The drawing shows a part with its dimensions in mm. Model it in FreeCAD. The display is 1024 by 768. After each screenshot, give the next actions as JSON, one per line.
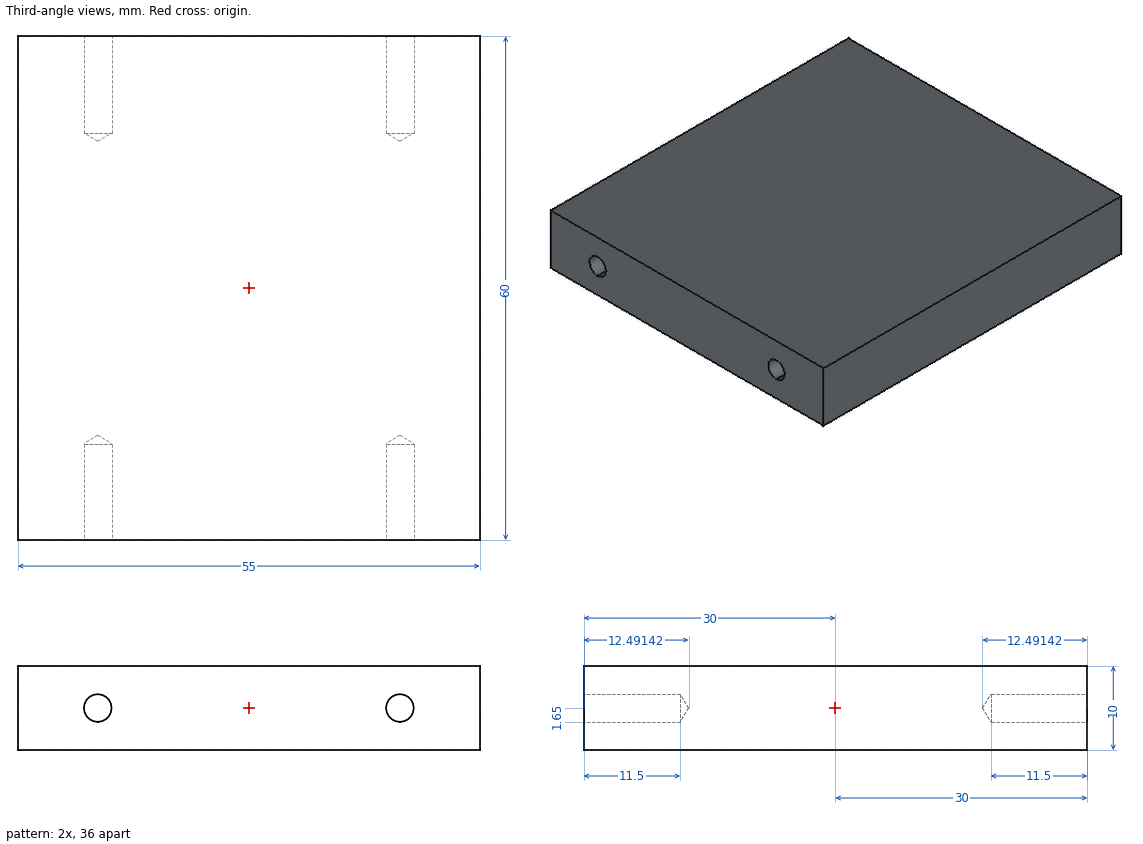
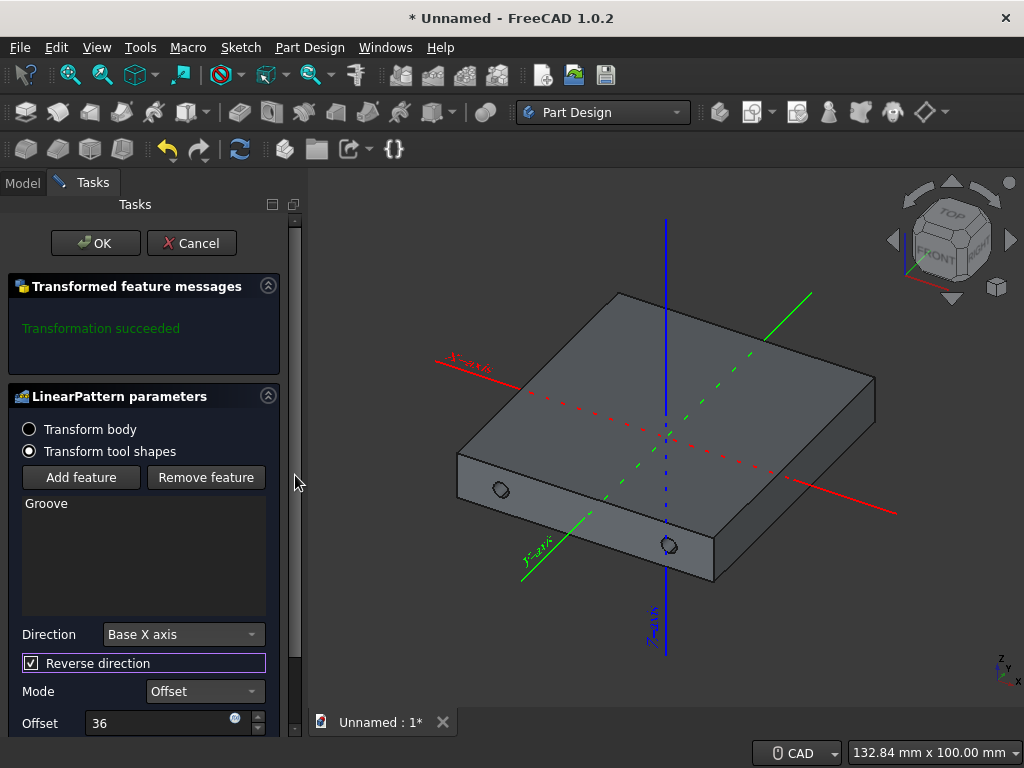
{"action": "left_click", "coordinate": [96, 243]}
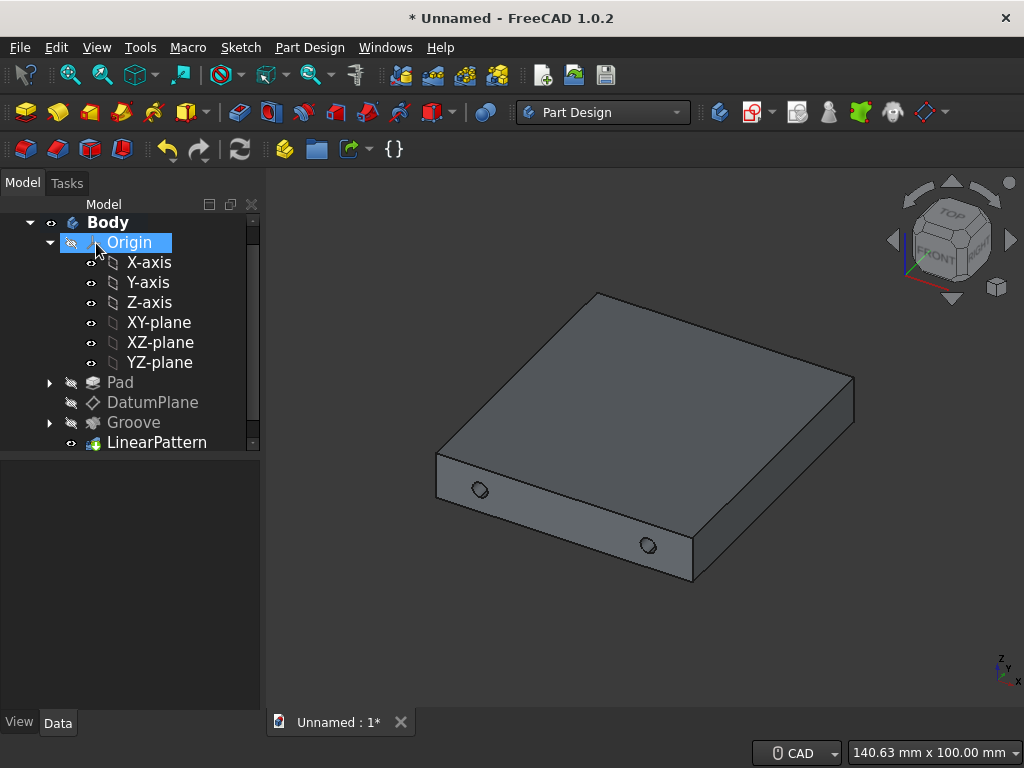
{"action": "left_click", "coordinate": [116, 423]}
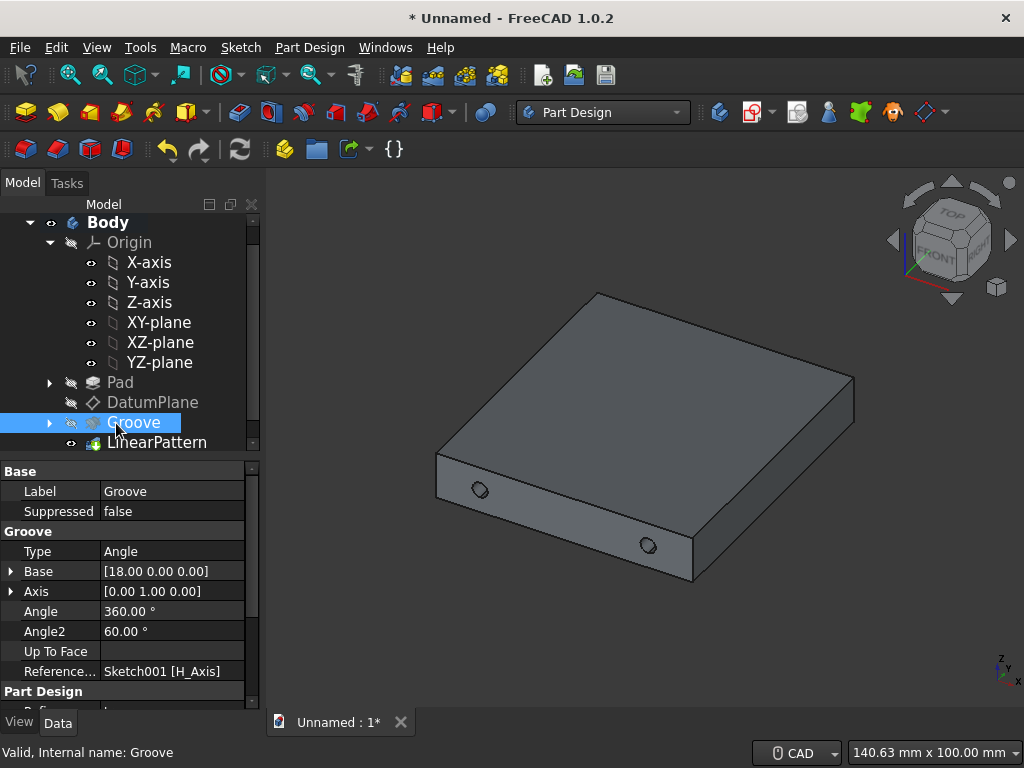
{"action": "left_click", "coordinate": [402, 76]}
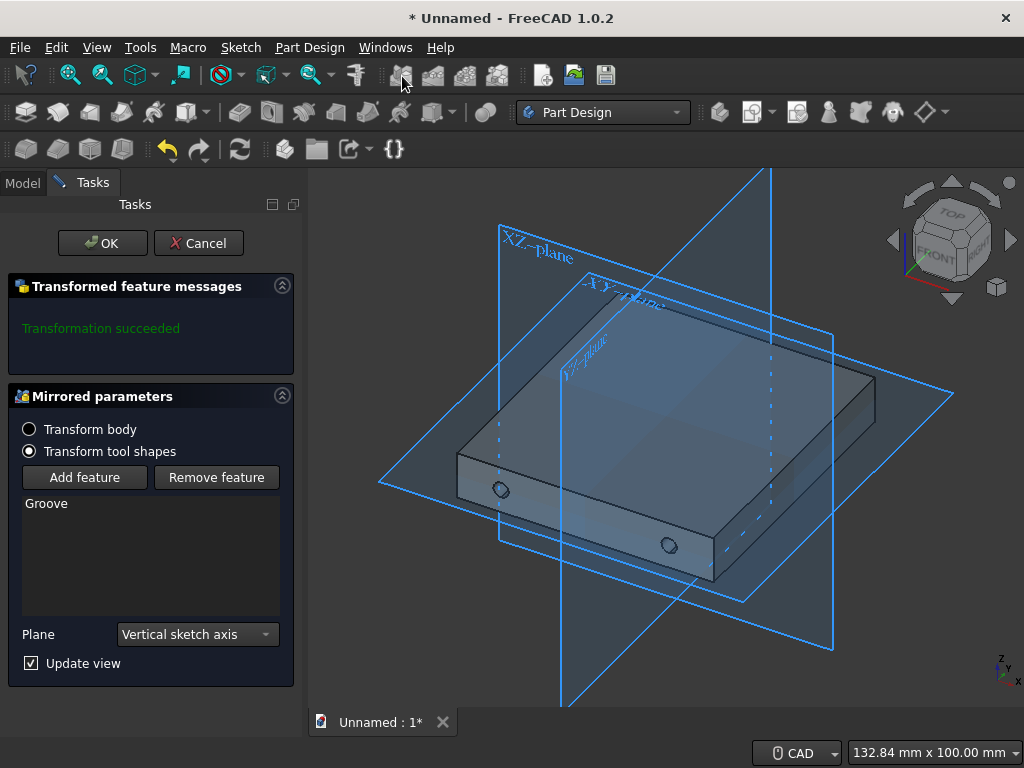
{"action": "left_click", "coordinate": [198, 634]}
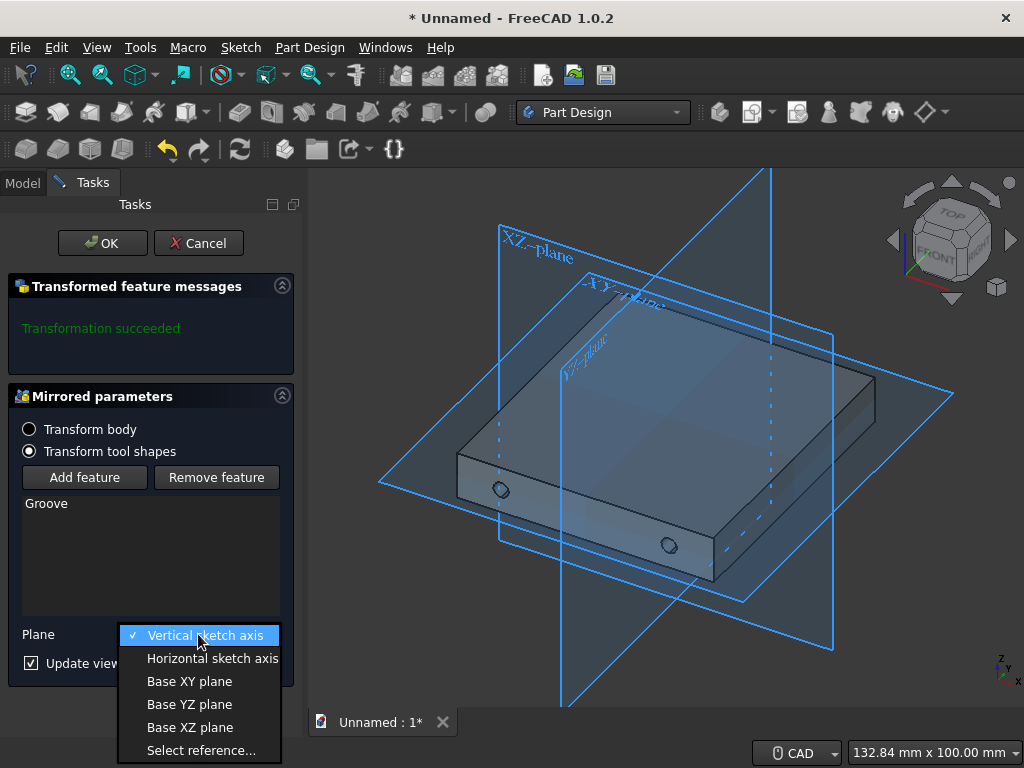
{"action": "left_click", "coordinate": [198, 728]}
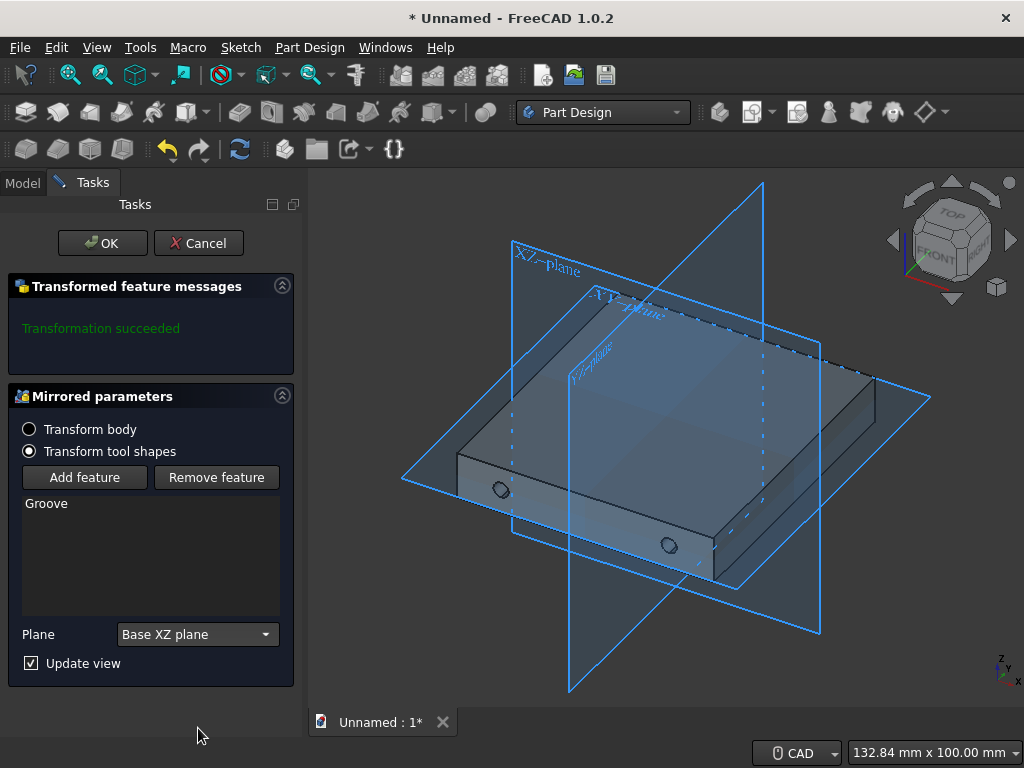
{"action": "left_click", "coordinate": [103, 243]}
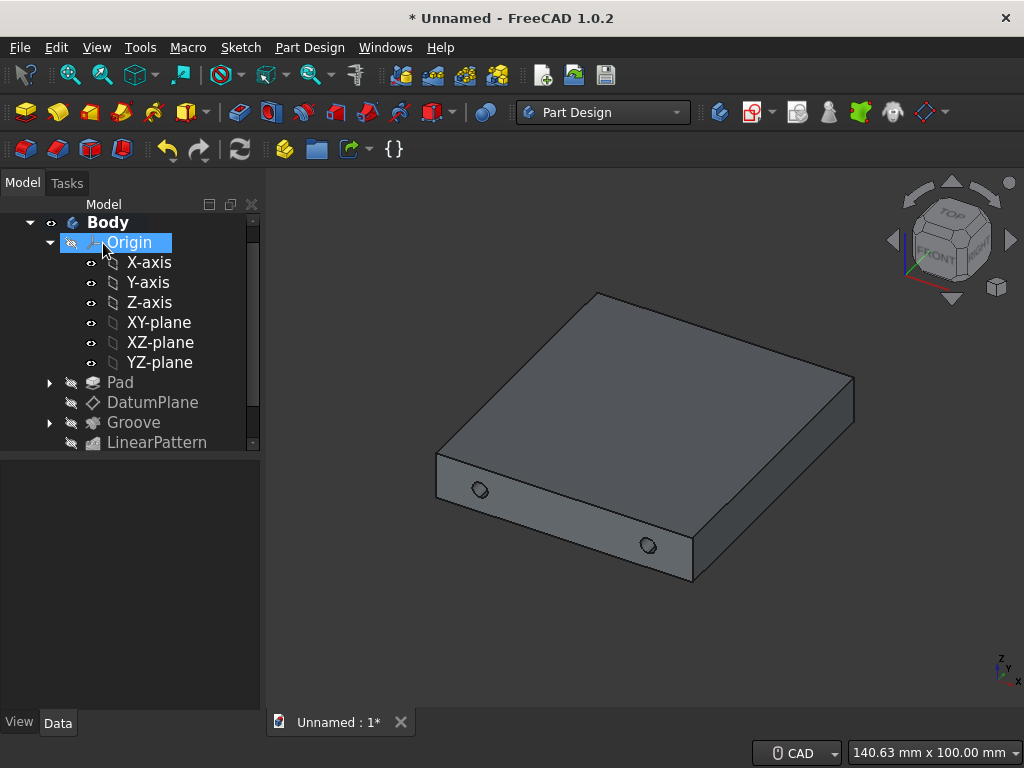
{"action": "left_click", "coordinate": [136, 363]}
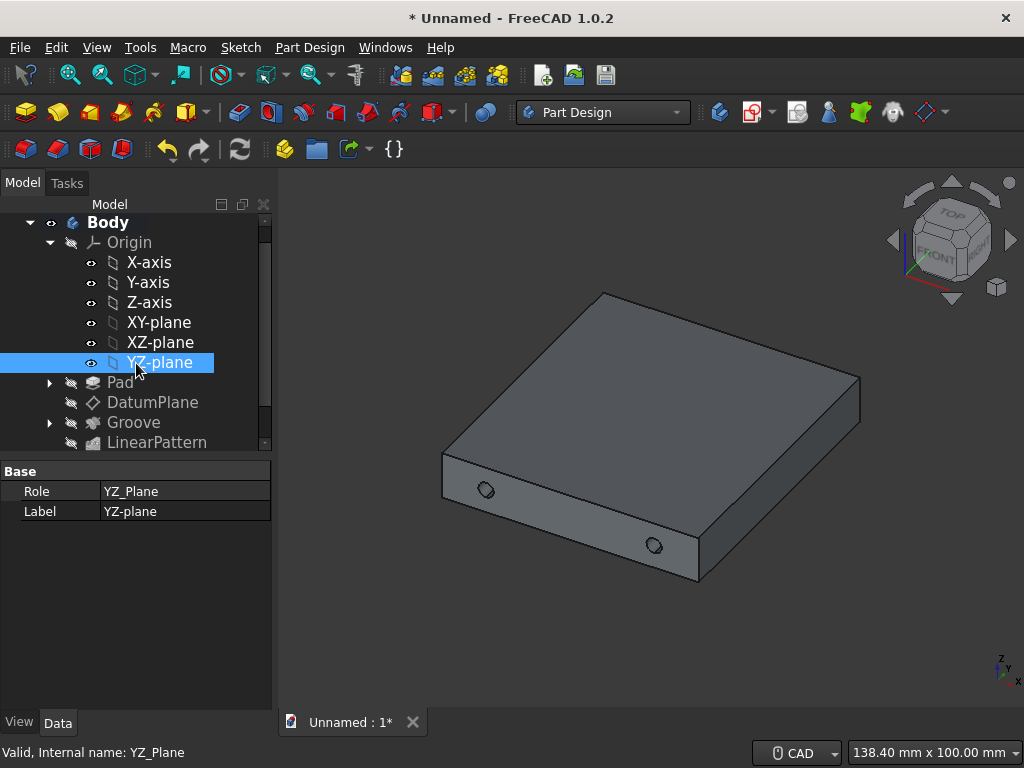
{"action": "left_click", "coordinate": [926, 112]}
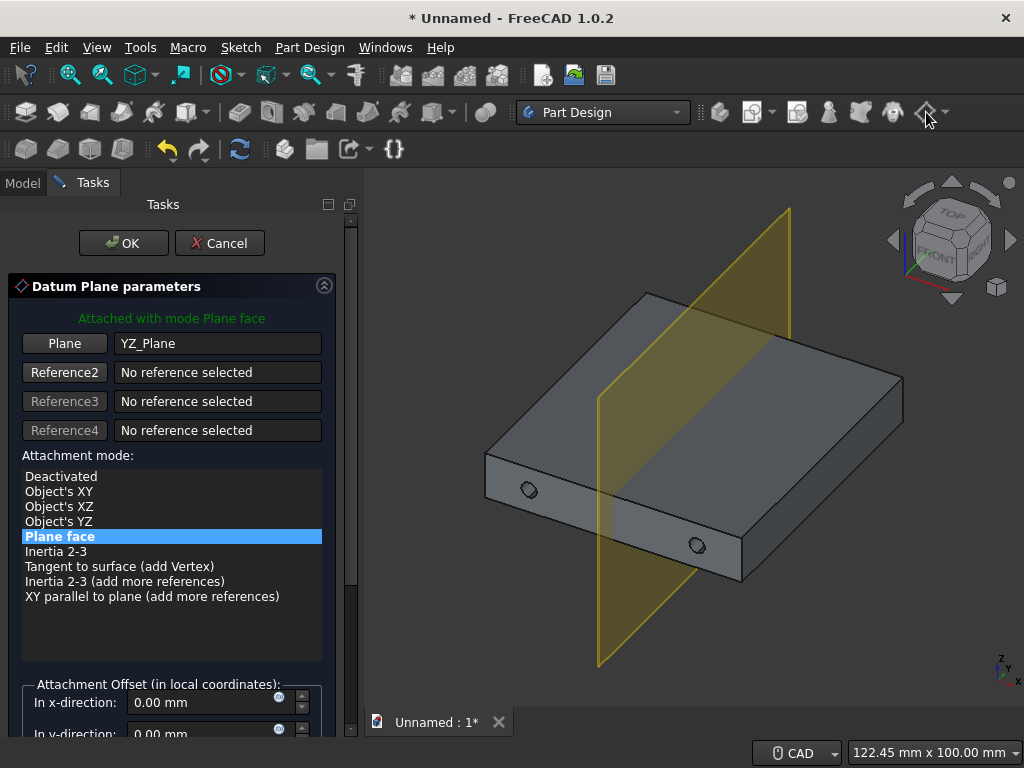
{"action": "scroll", "coordinate": [351, 475], "scroll_direction": "down", "scroll_amount": 2}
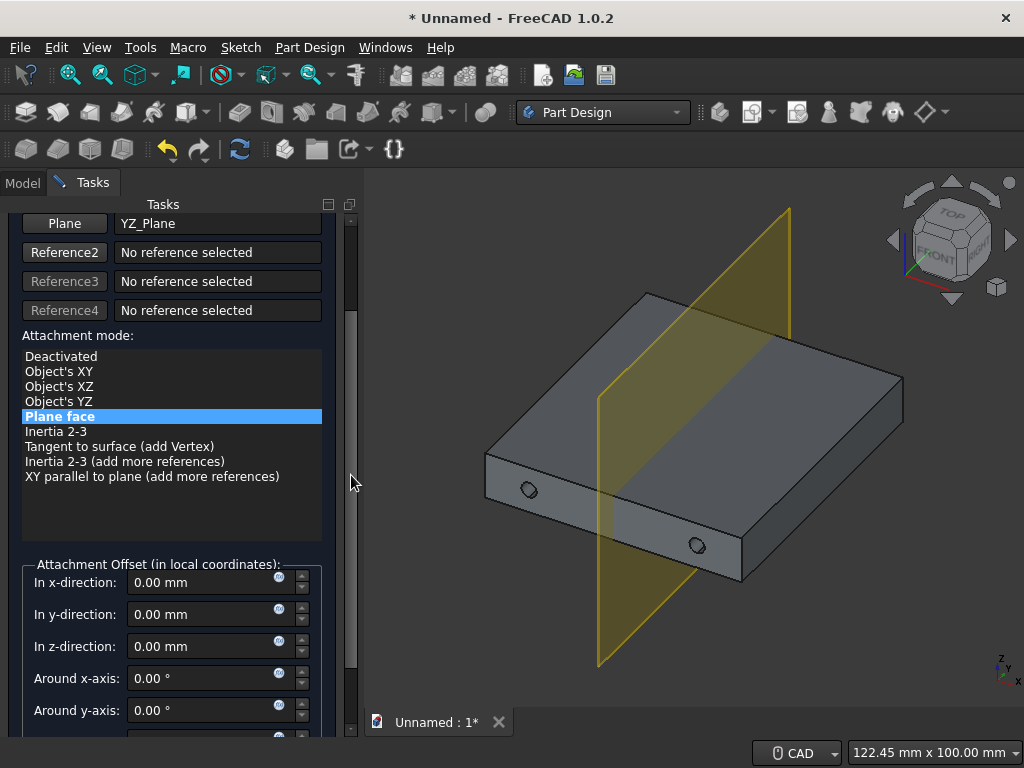
{"action": "triple_click", "coordinate": [210, 646]}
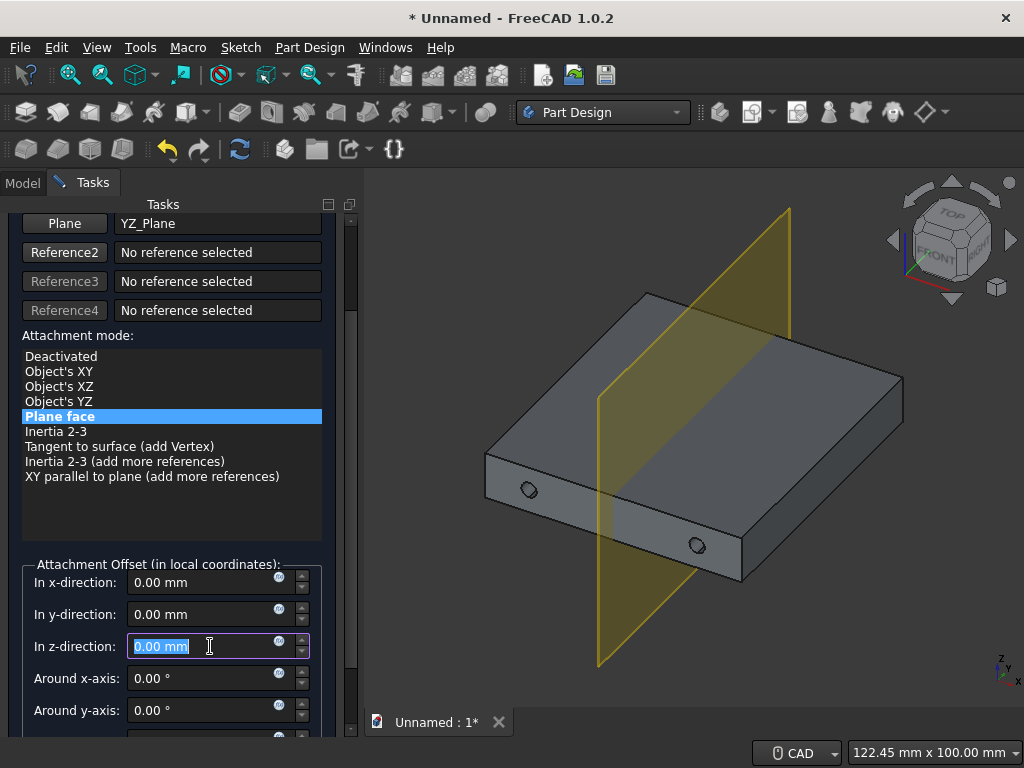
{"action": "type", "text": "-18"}
{"action": "key", "text": "Tab"}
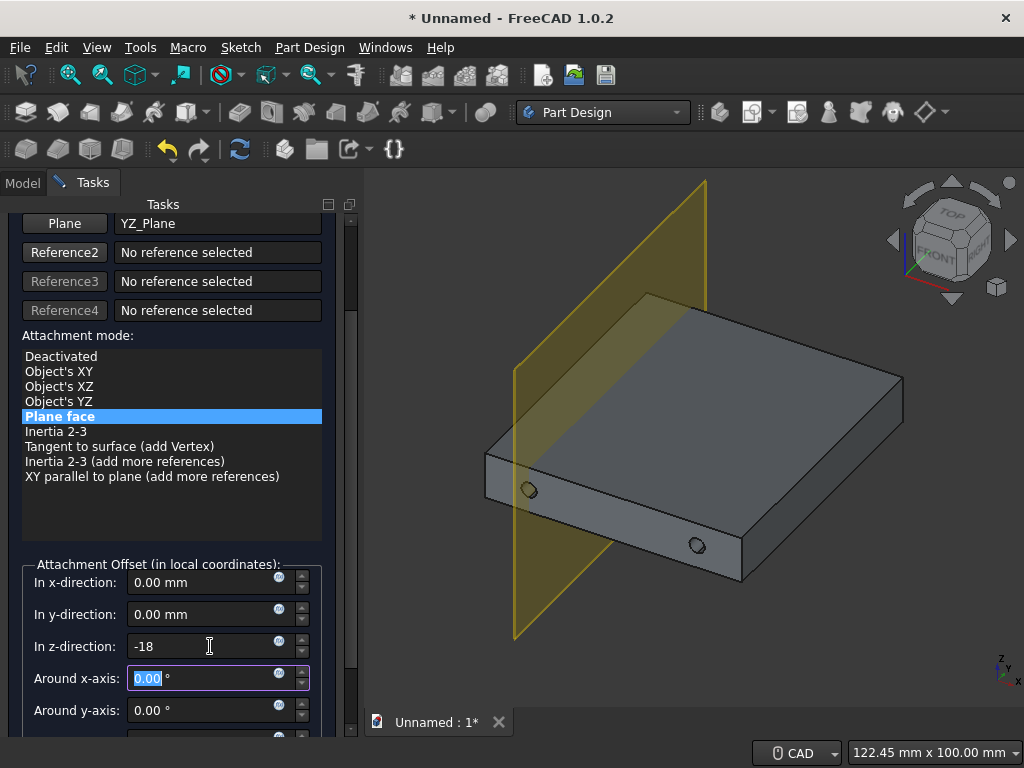
{"action": "scroll", "coordinate": [351, 475], "scroll_direction": "up", "scroll_amount": 3}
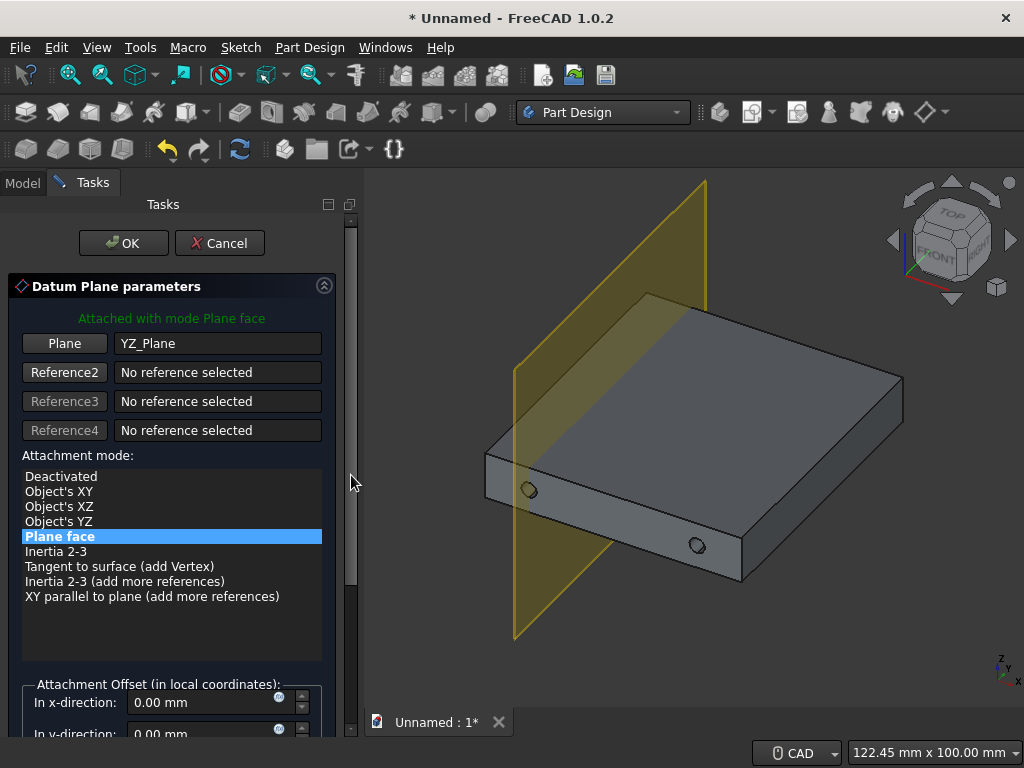
{"action": "left_click", "coordinate": [124, 243]}